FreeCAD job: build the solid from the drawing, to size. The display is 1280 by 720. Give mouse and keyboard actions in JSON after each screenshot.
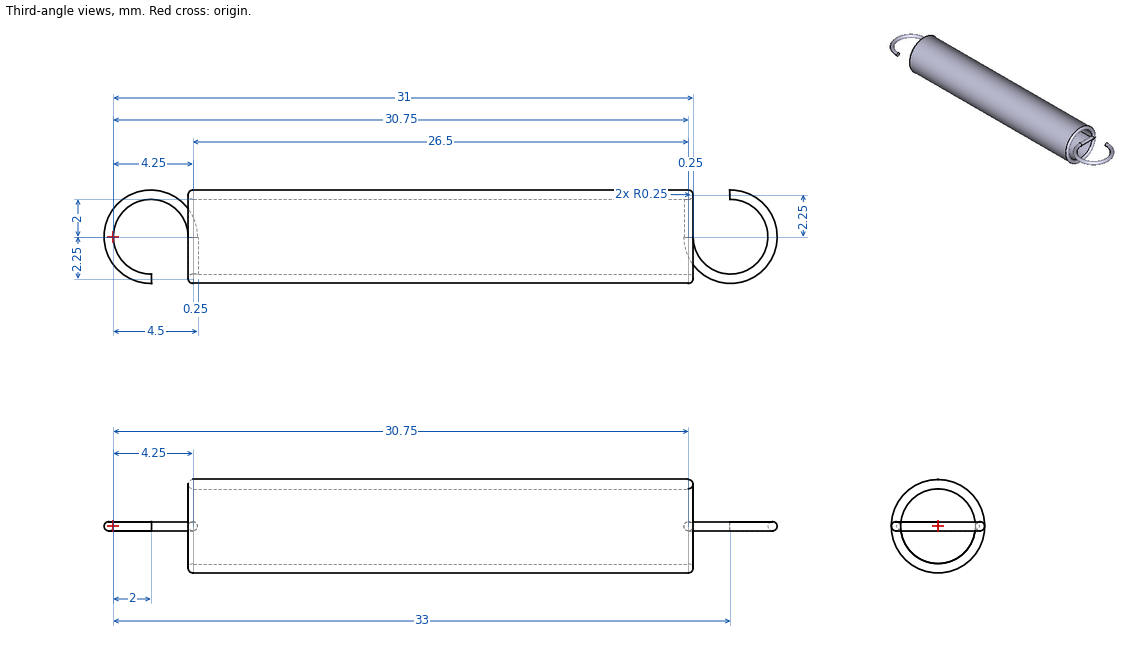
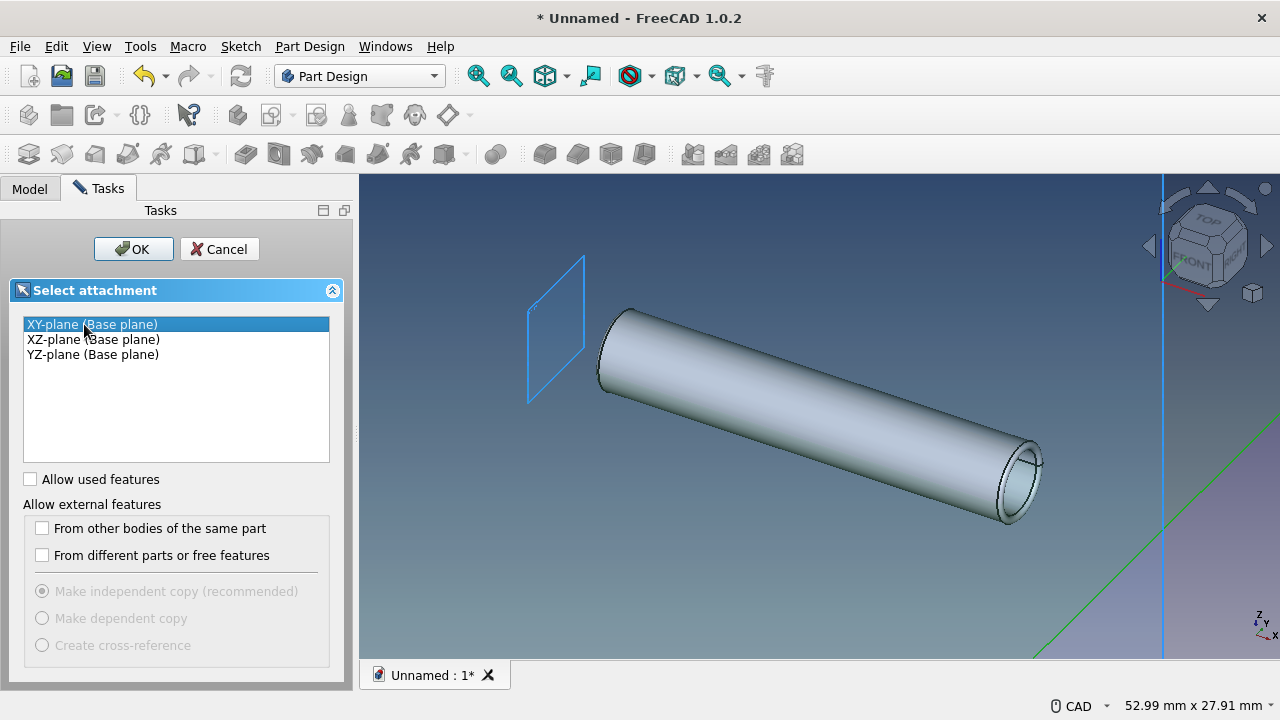
{"action": "left_click", "coordinate": [134, 249]}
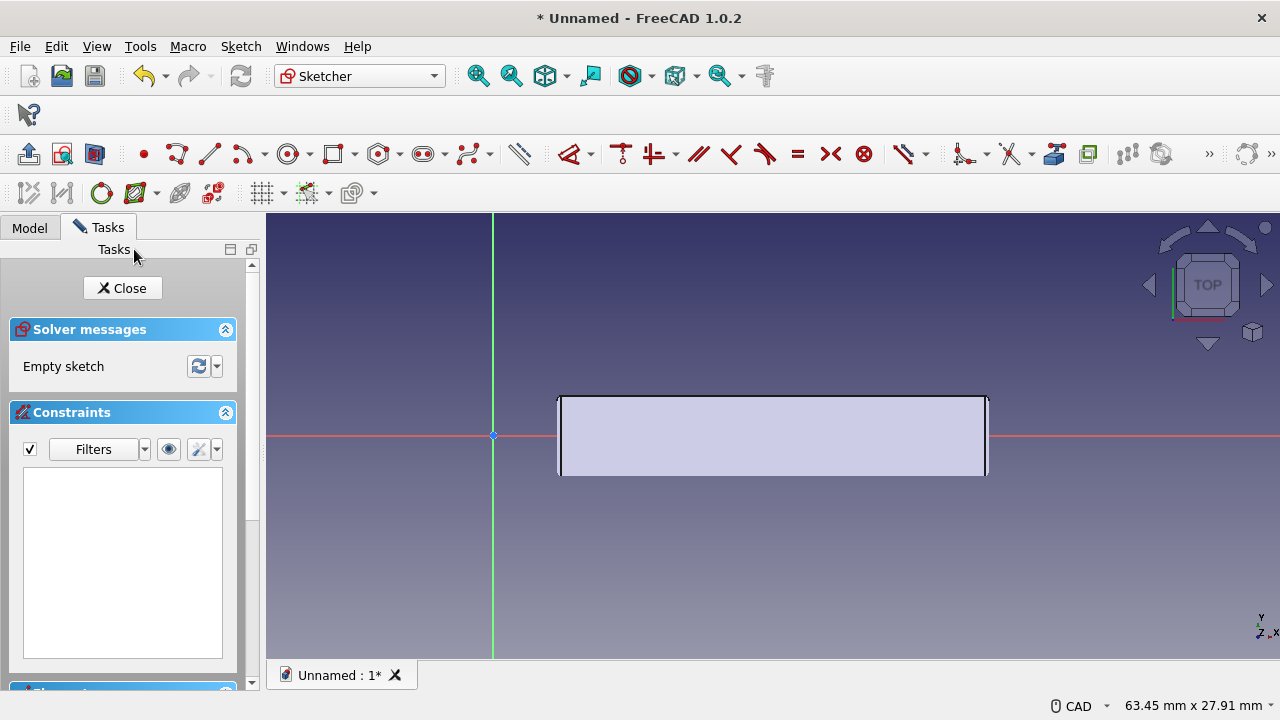
{"action": "key", "text": "q s"}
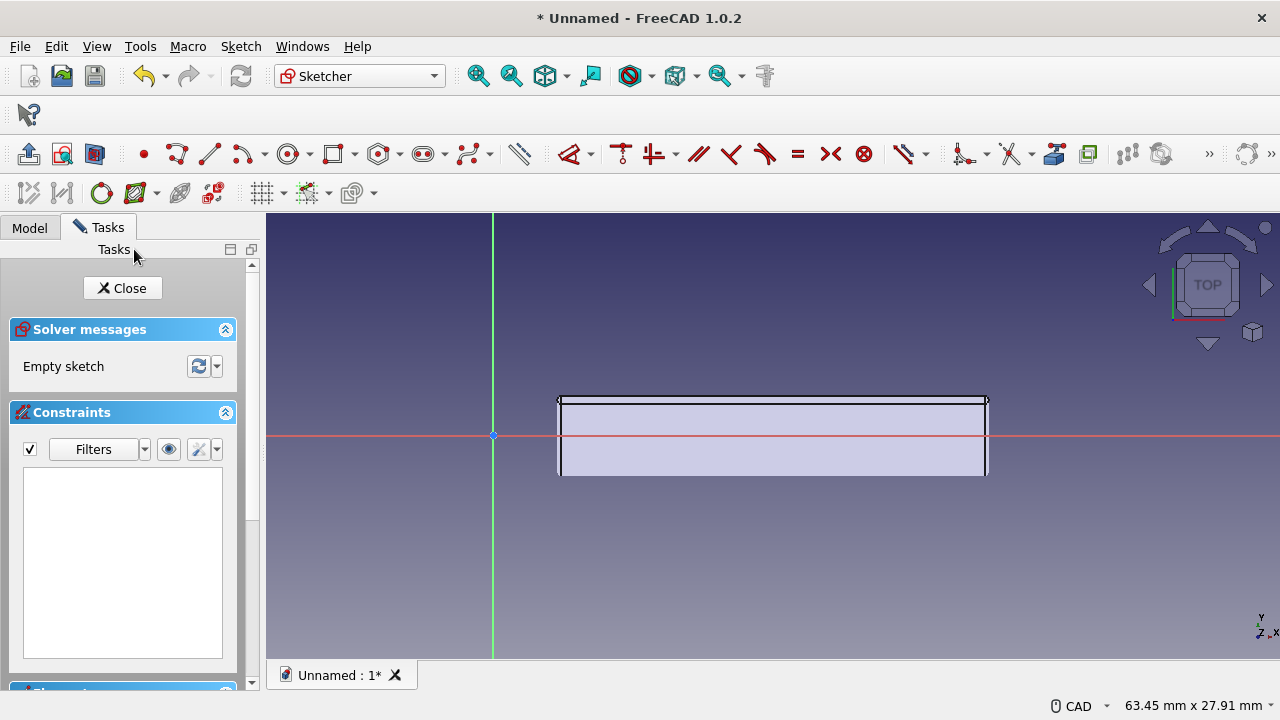
{"action": "scroll", "coordinate": [1058, 404], "scroll_direction": "up", "scroll_amount": 8}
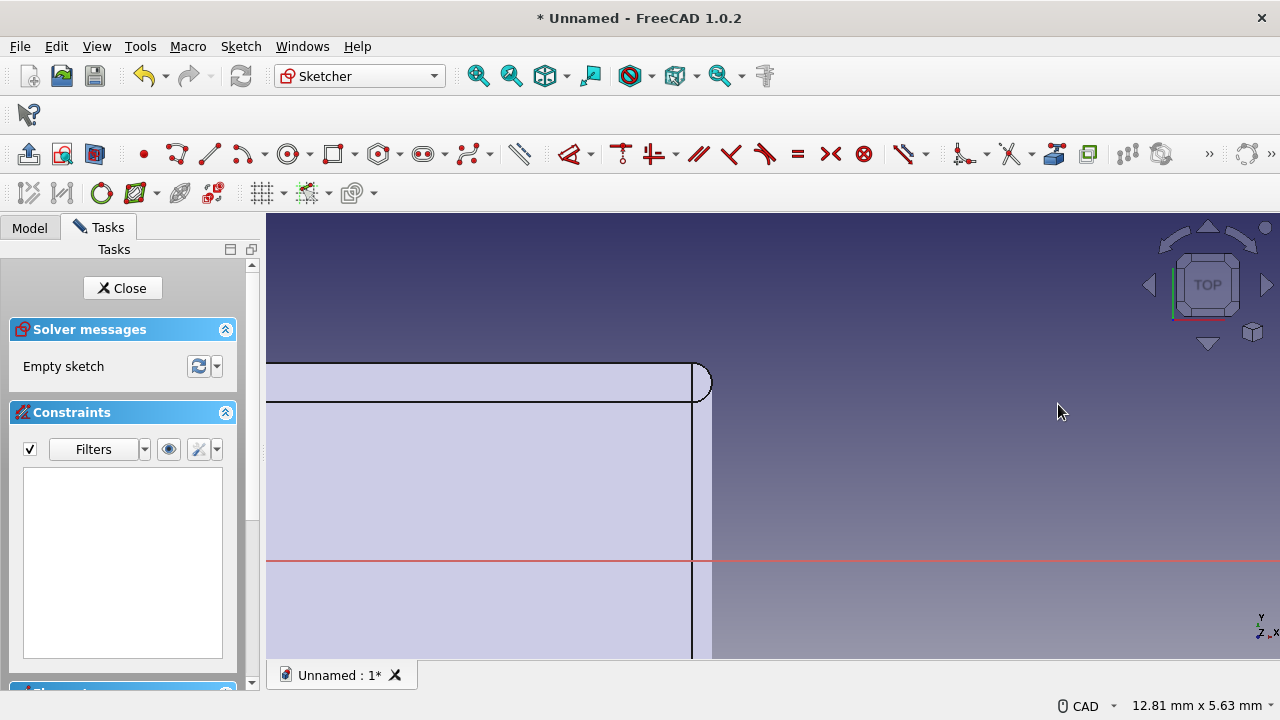
{"action": "left_click", "coordinate": [332, 154]}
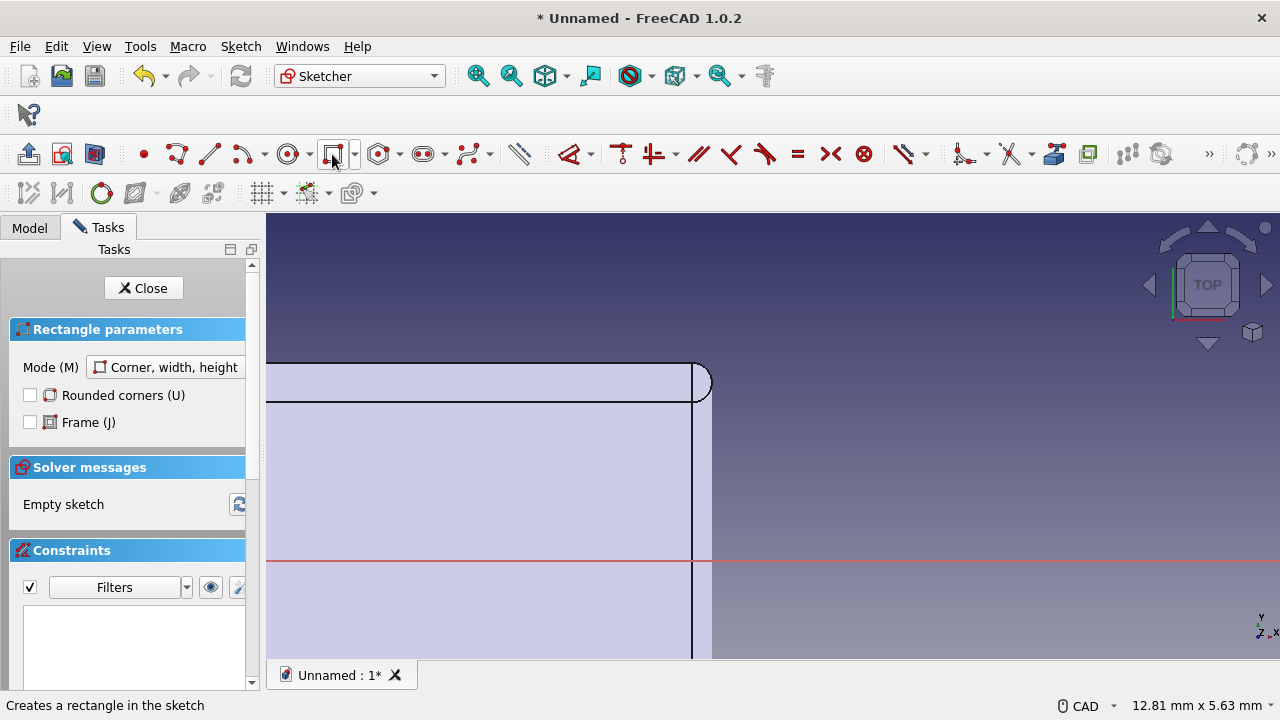
{"action": "left_click", "coordinate": [692, 383]}
{"action": "left_click", "coordinate": [712, 561]}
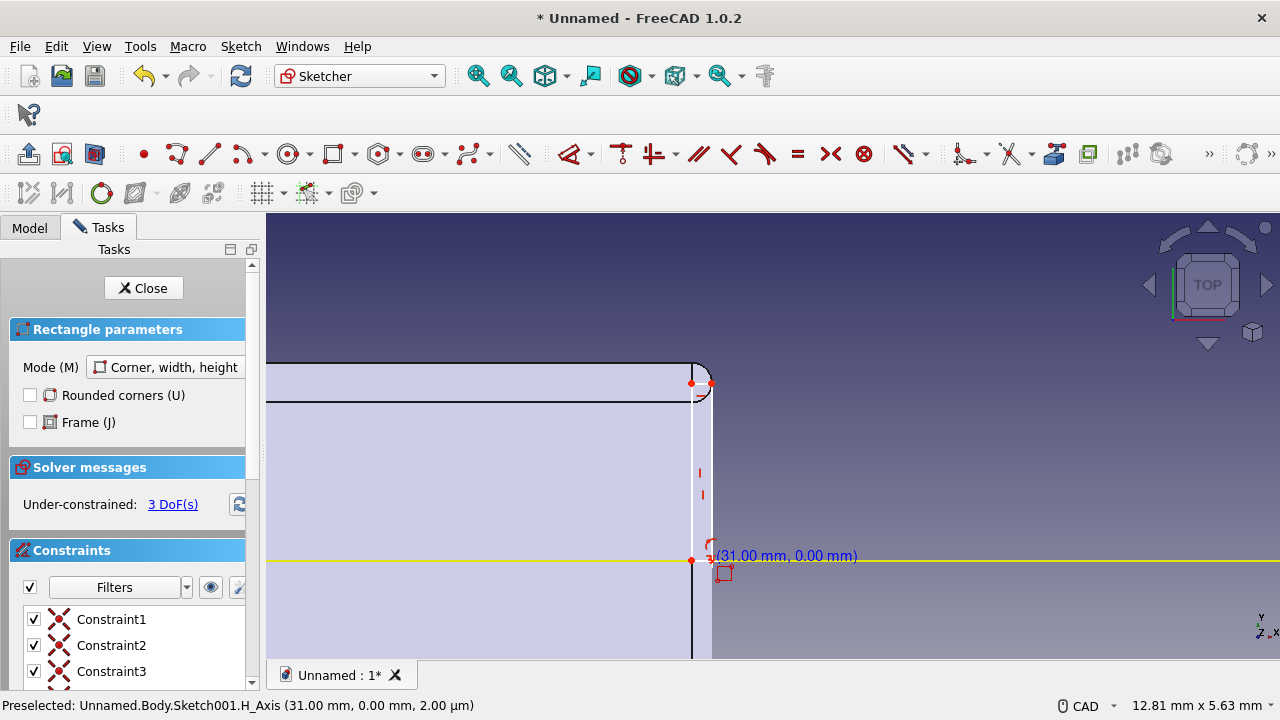
{"action": "key", "text": "g l"}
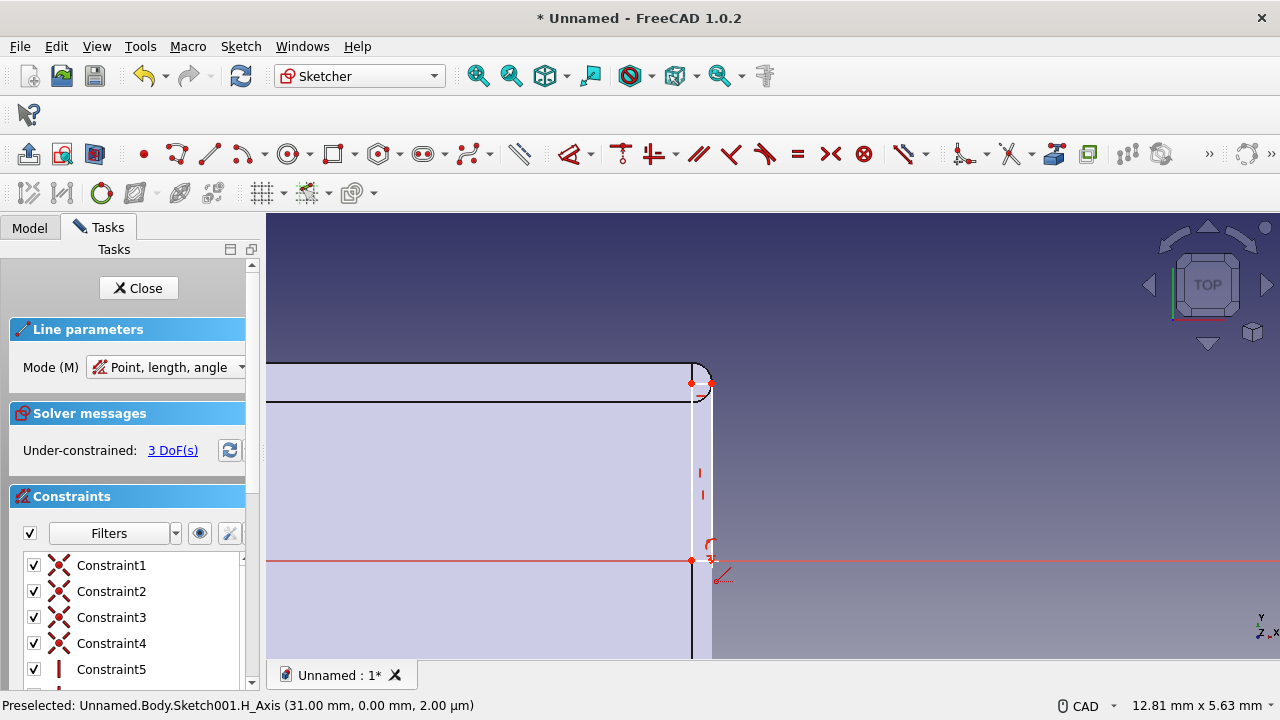
{"action": "left_click", "coordinate": [692, 365]}
{"action": "left_click", "coordinate": [692, 311]}
{"action": "key", "text": "Escape"}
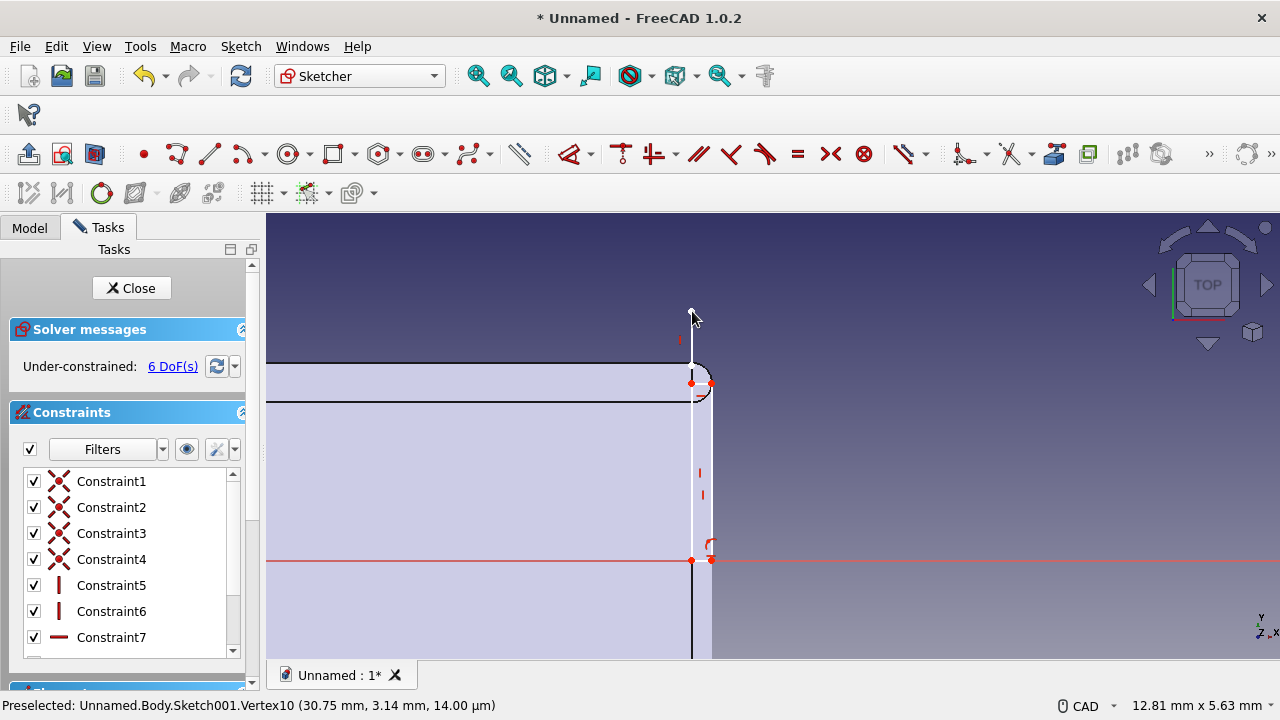
{"action": "left_click", "coordinate": [692, 350]}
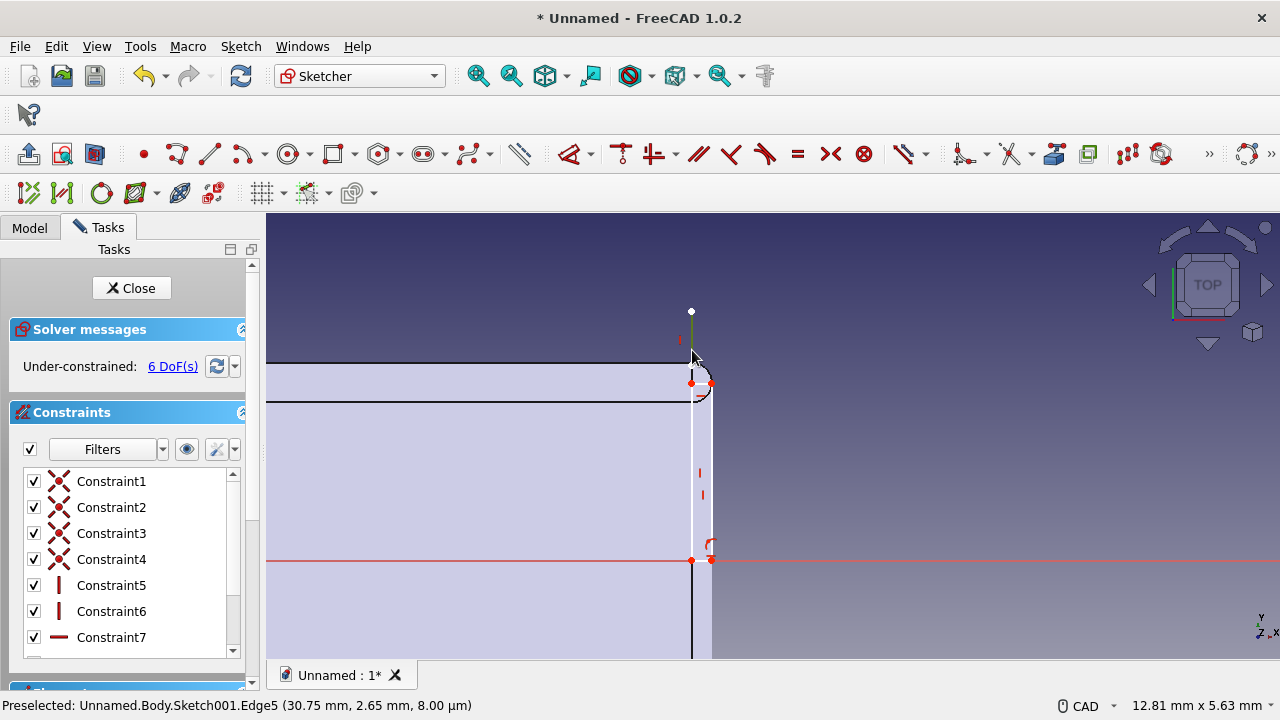
{"action": "key", "text": "g n"}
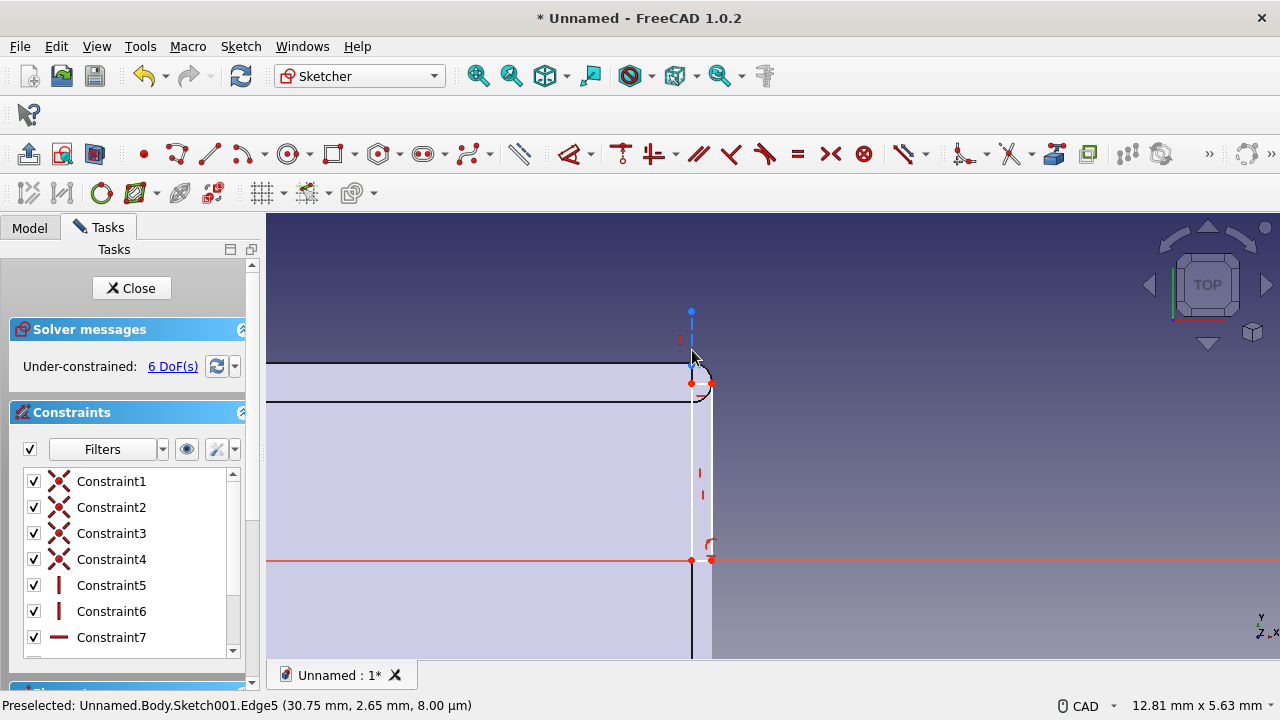
{"action": "key", "text": "d"}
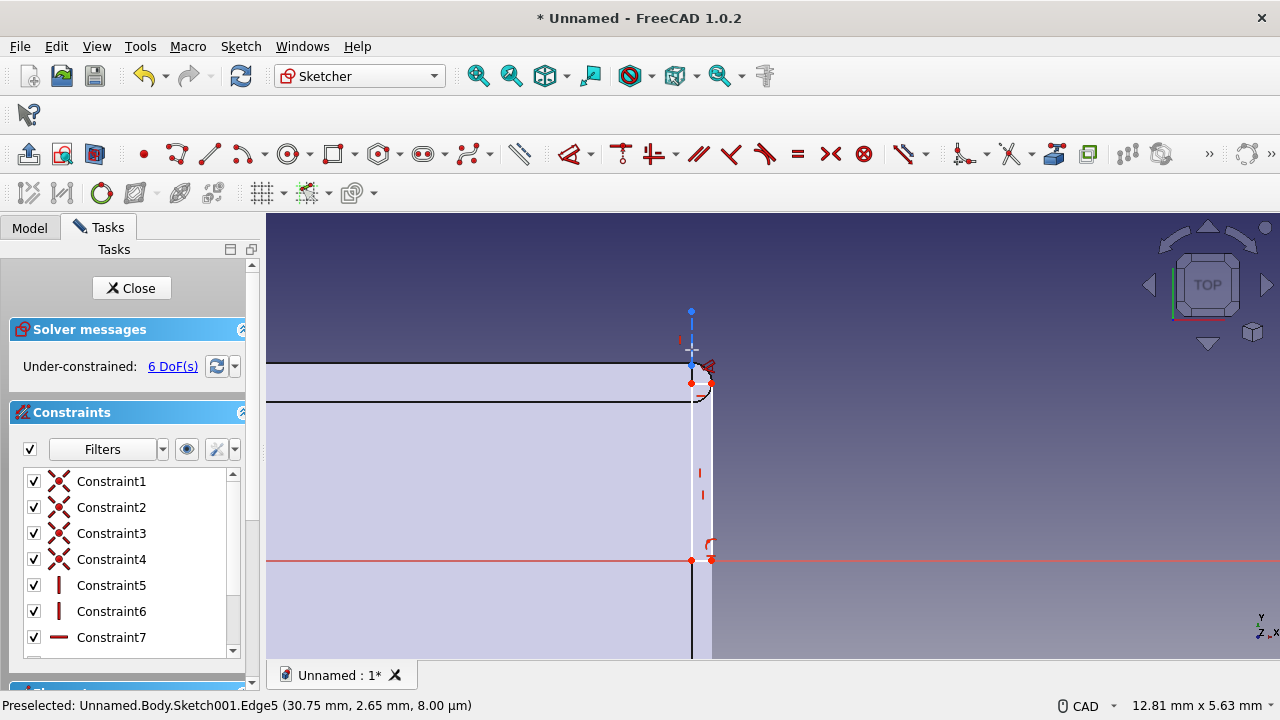
{"action": "left_click", "coordinate": [712, 561]}
{"action": "left_click", "coordinate": [503, 595]}